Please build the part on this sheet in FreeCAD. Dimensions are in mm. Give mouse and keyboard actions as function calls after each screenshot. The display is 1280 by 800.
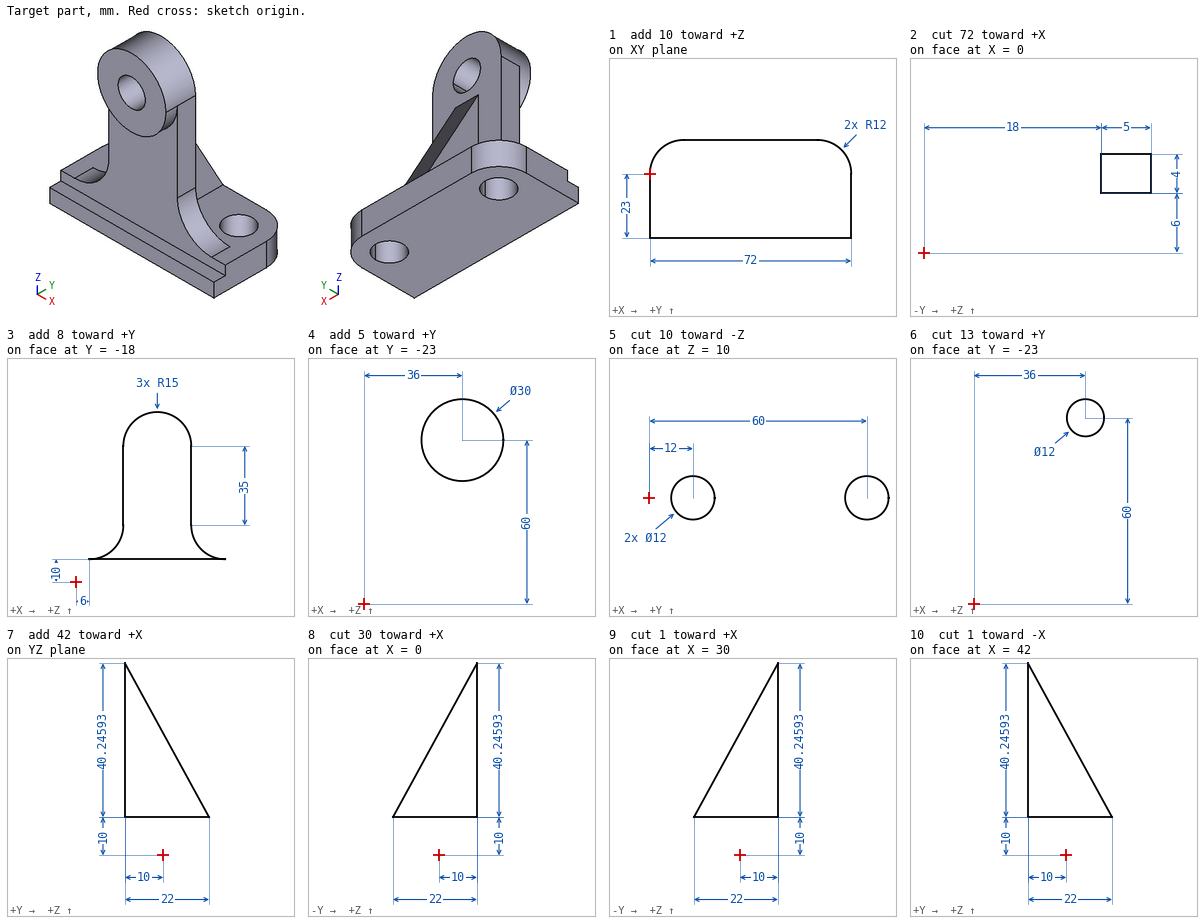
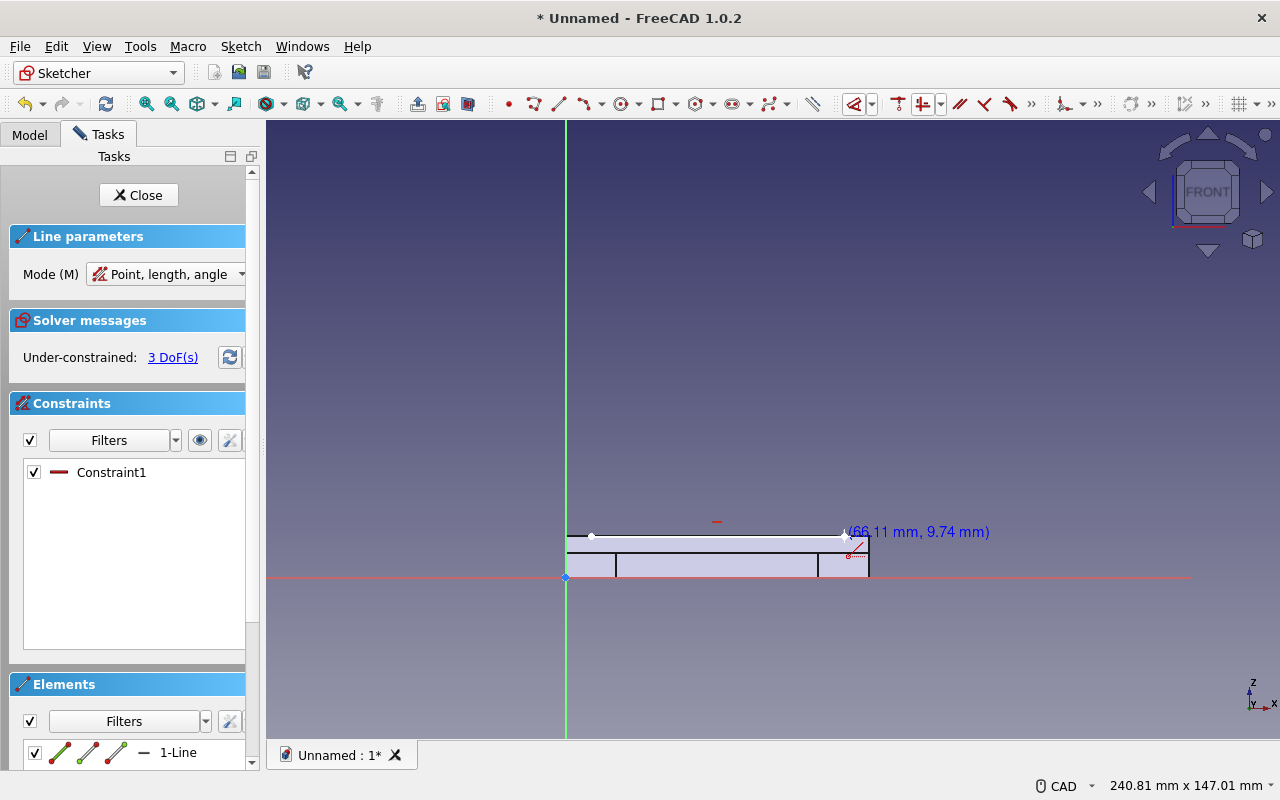
click(780, 473)
click(780, 325)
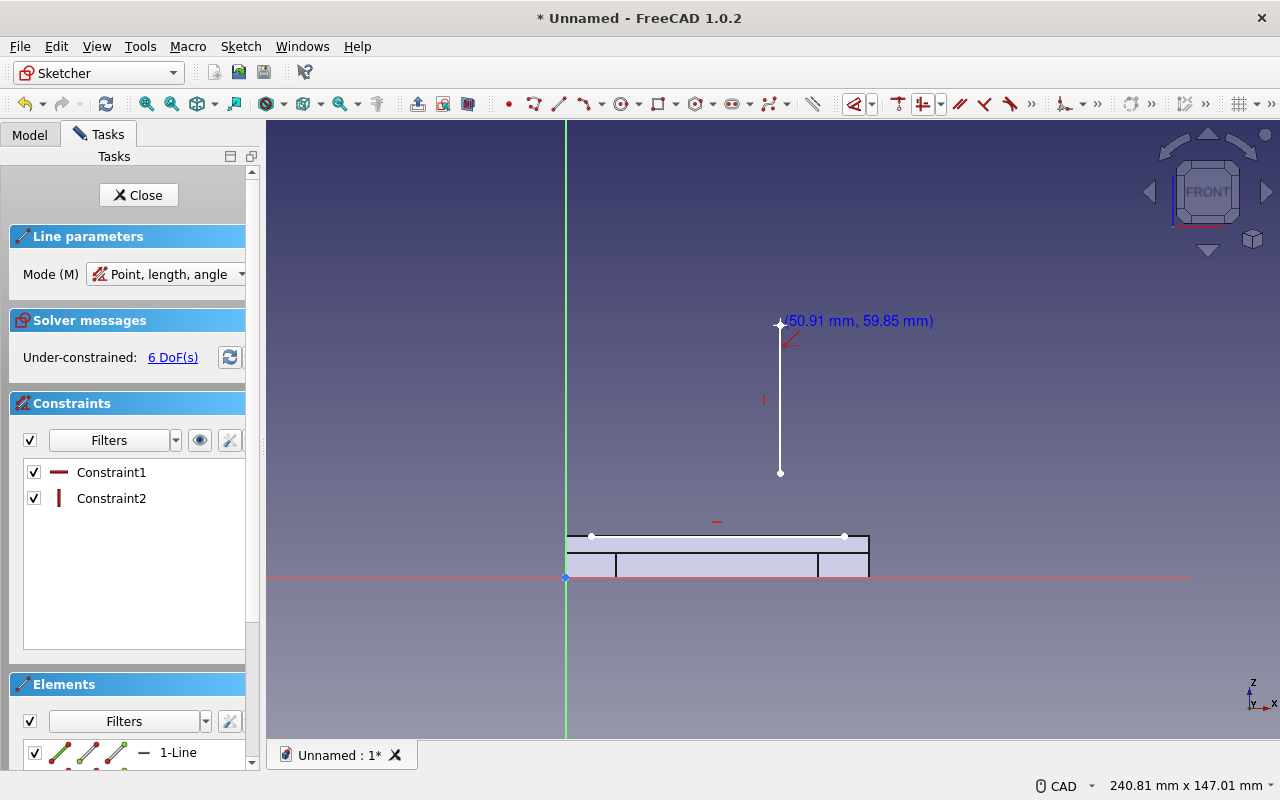
click(654, 325)
click(654, 473)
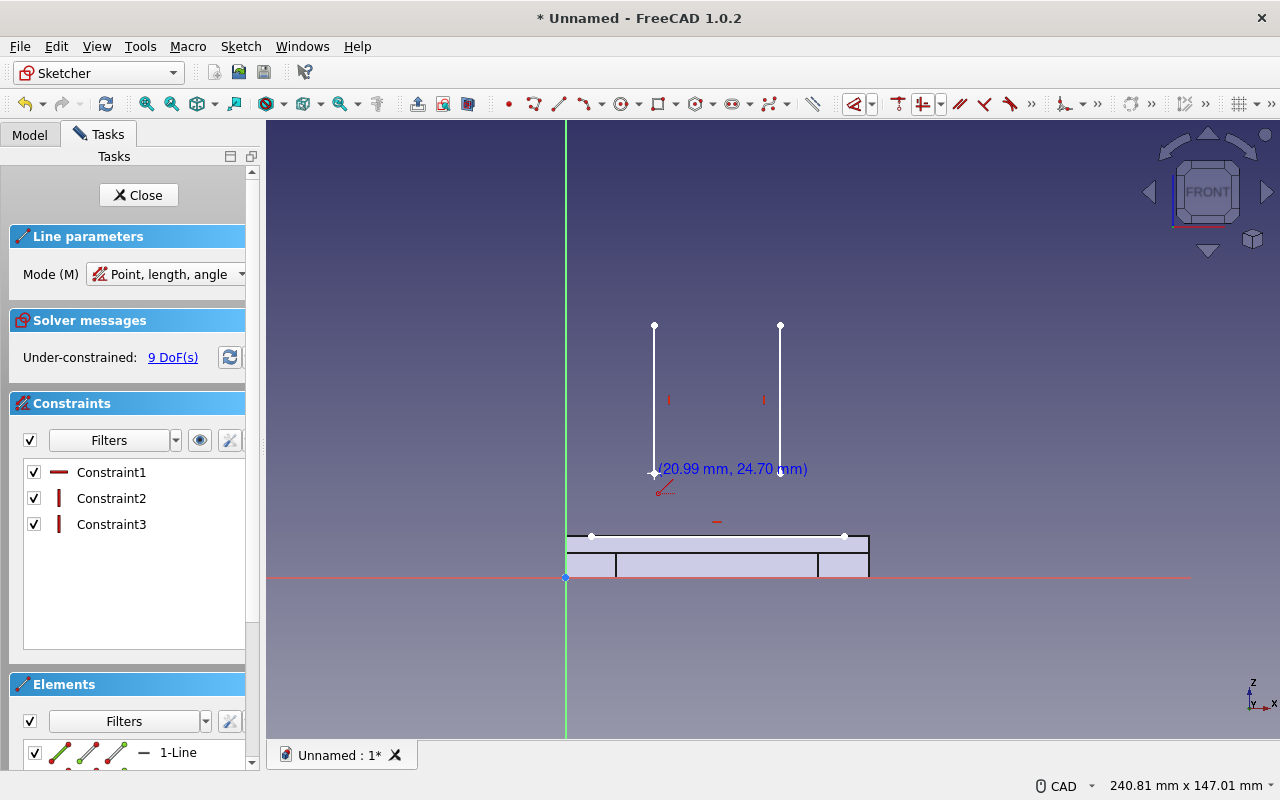
click(584, 104)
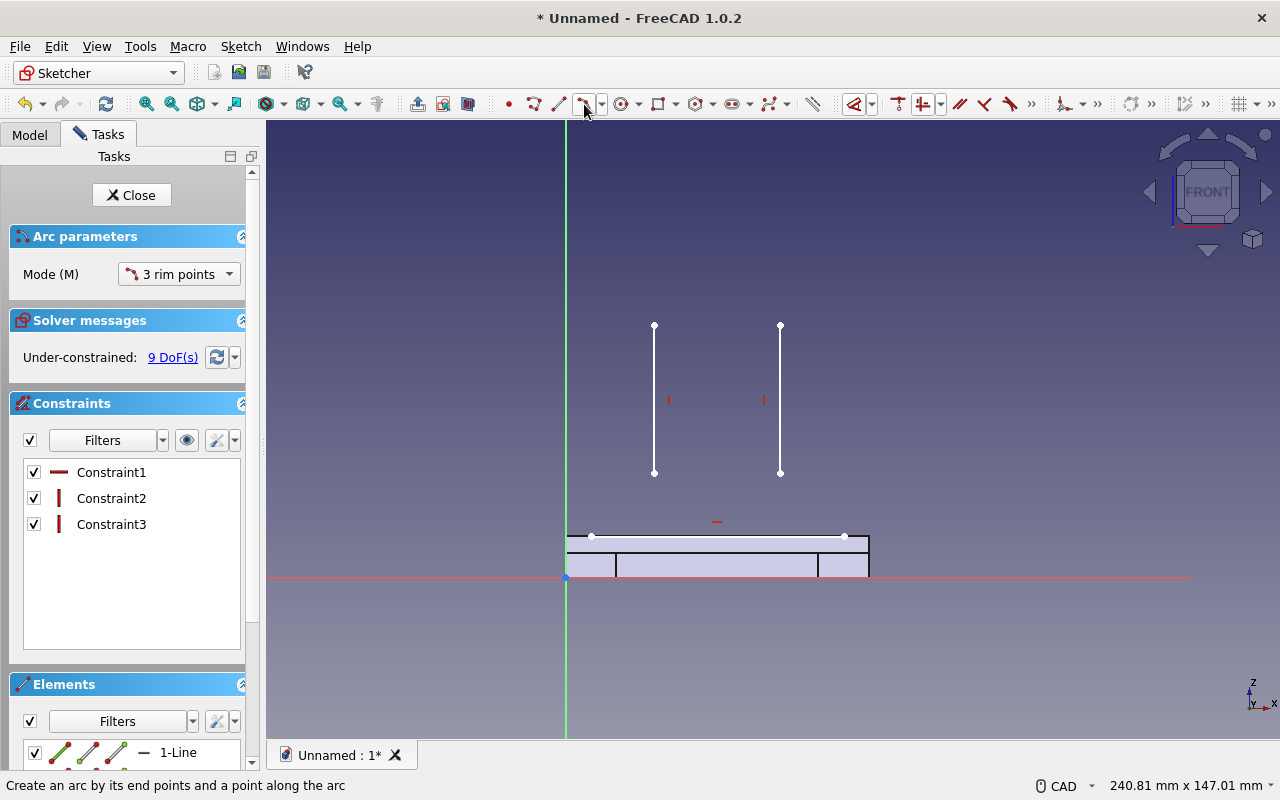
click(844, 537)
click(780, 474)
click(799, 517)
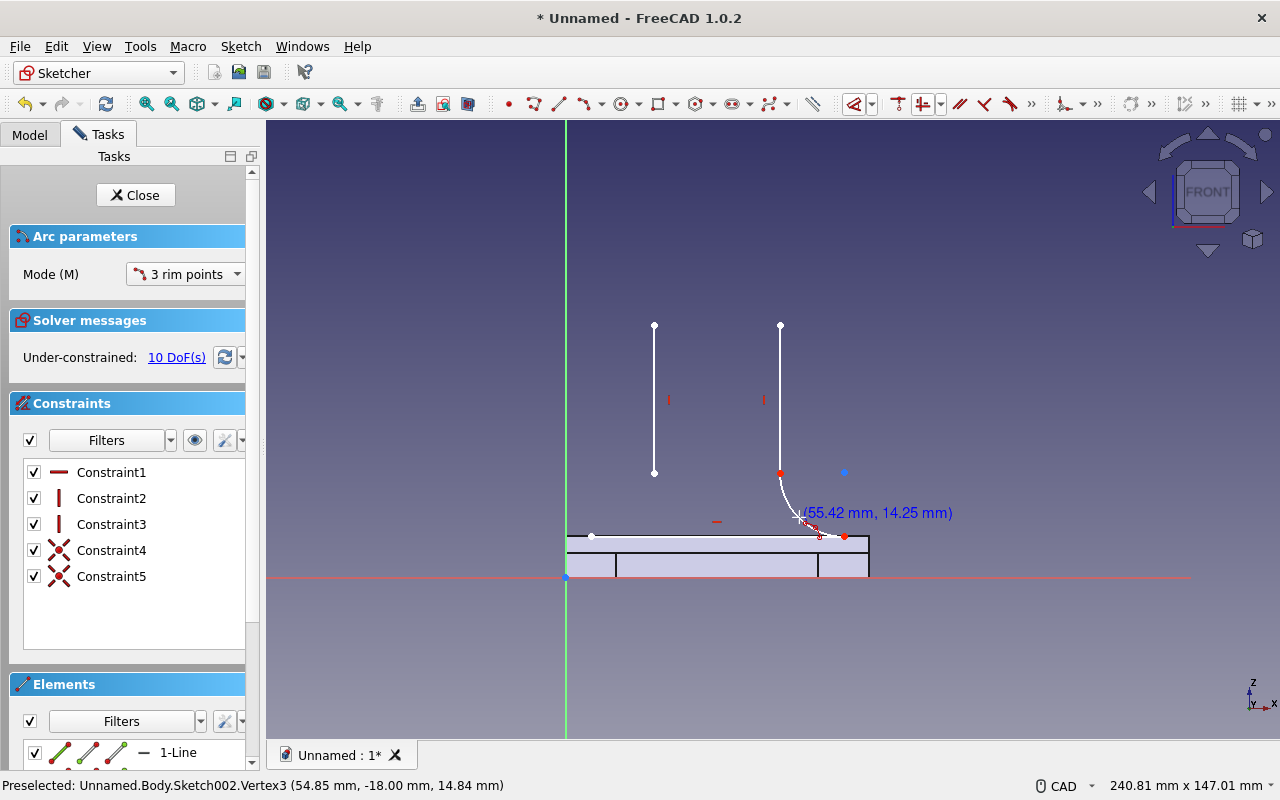
click(780, 326)
click(654, 326)
click(717, 262)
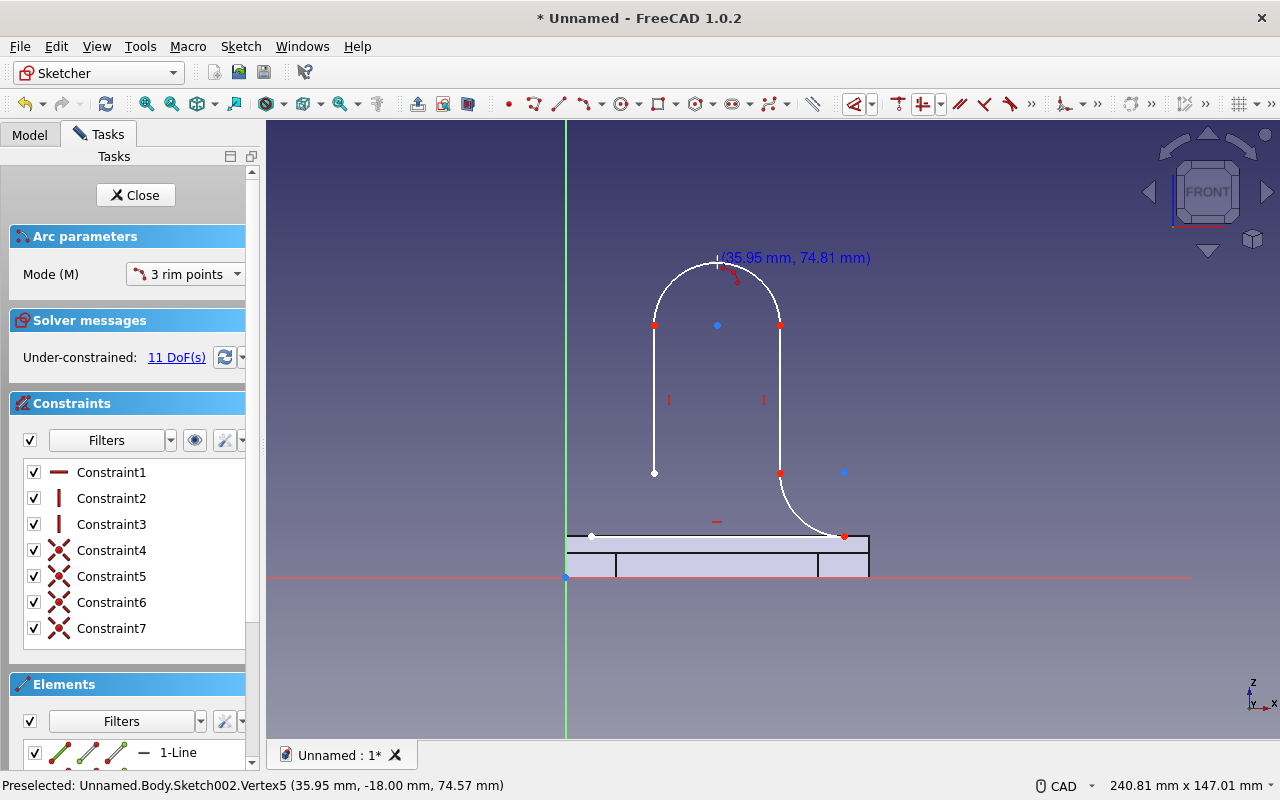
click(654, 474)
click(591, 537)
click(636, 517)
key(Escape)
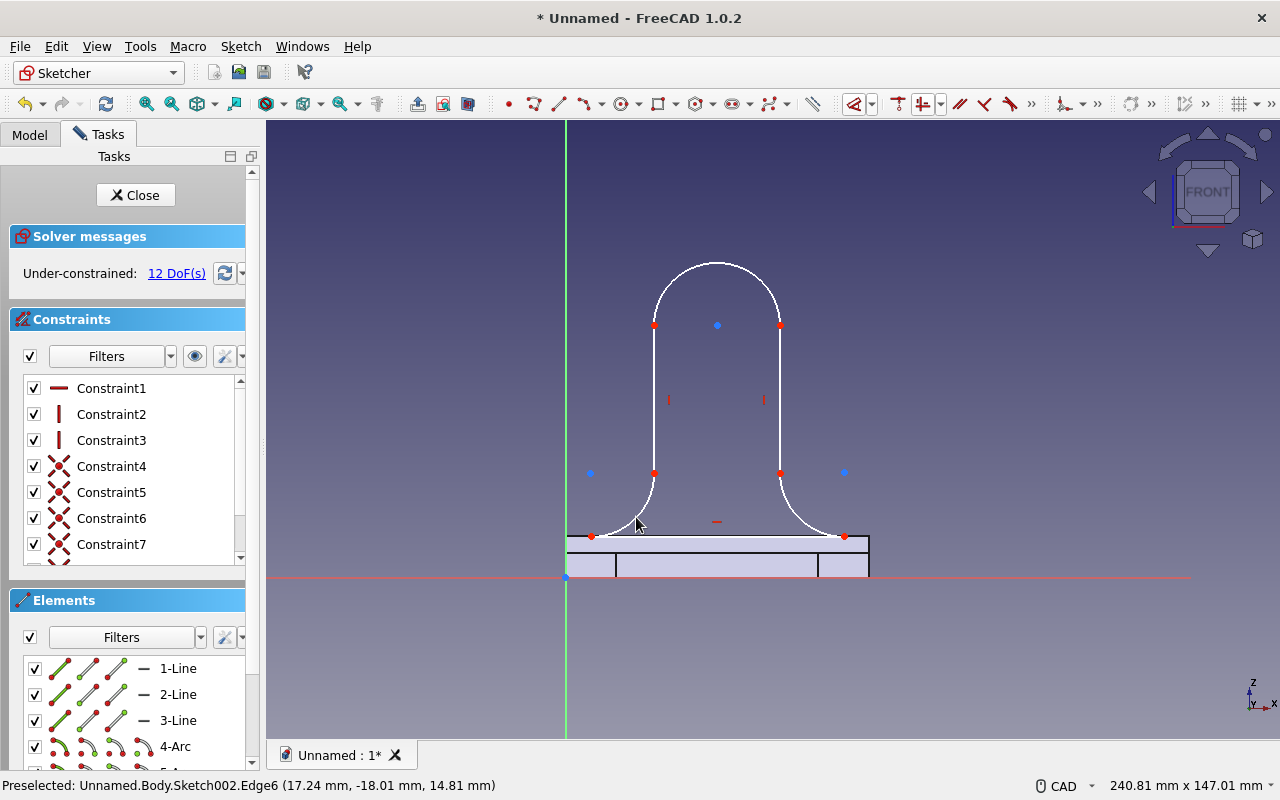
click(667, 537)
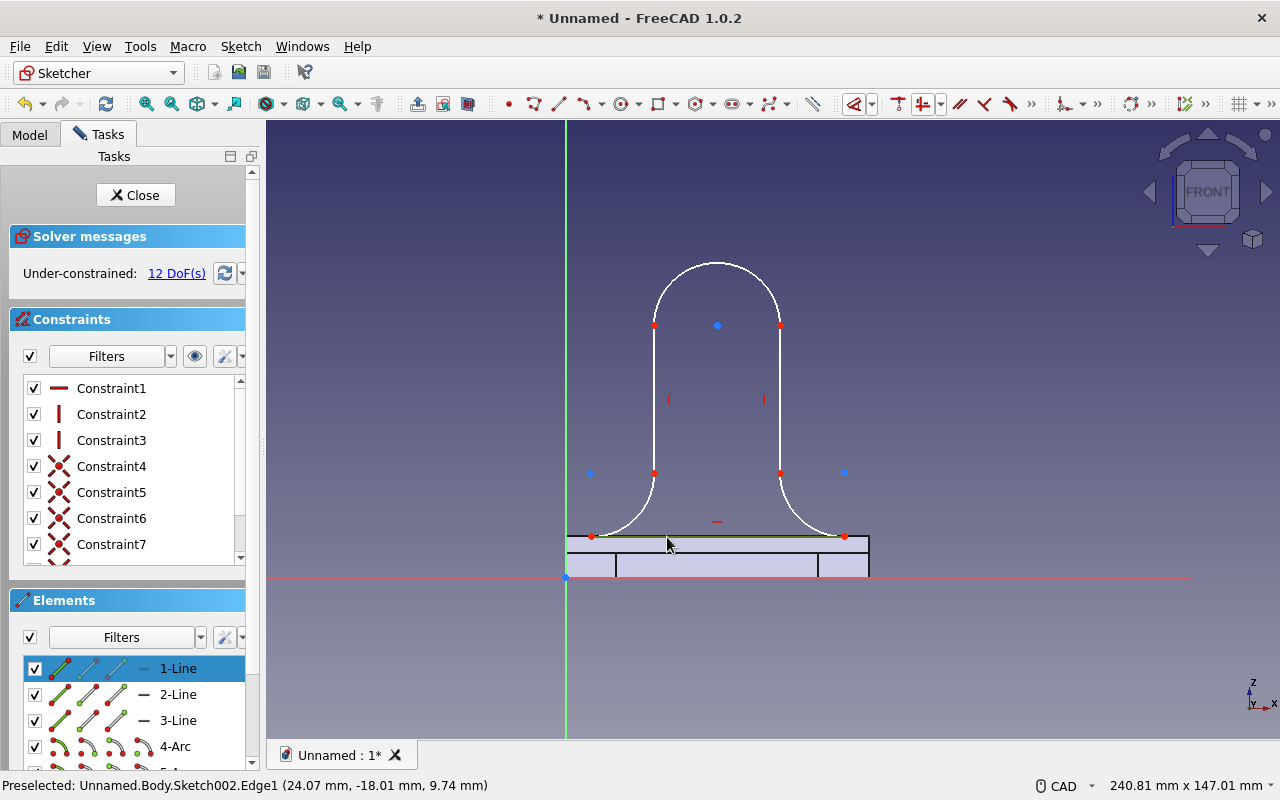
click(788, 503)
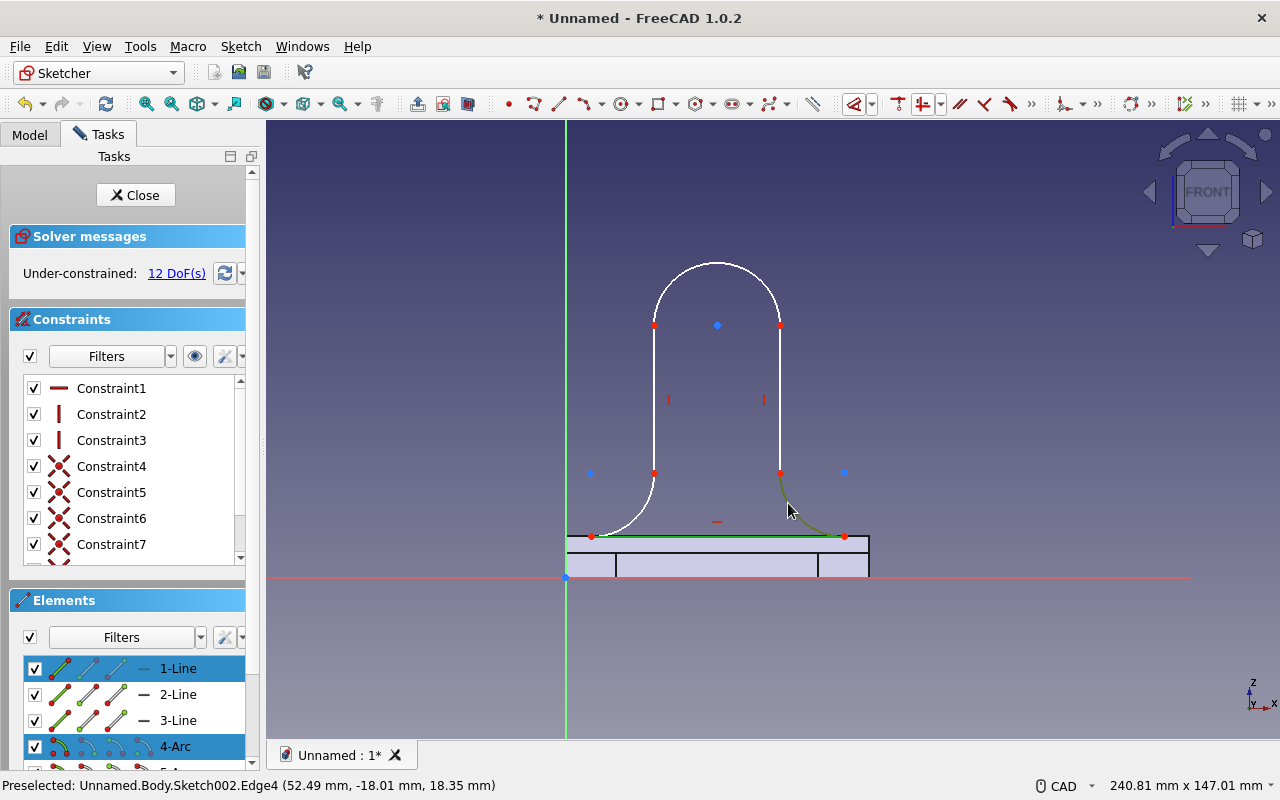
key(t)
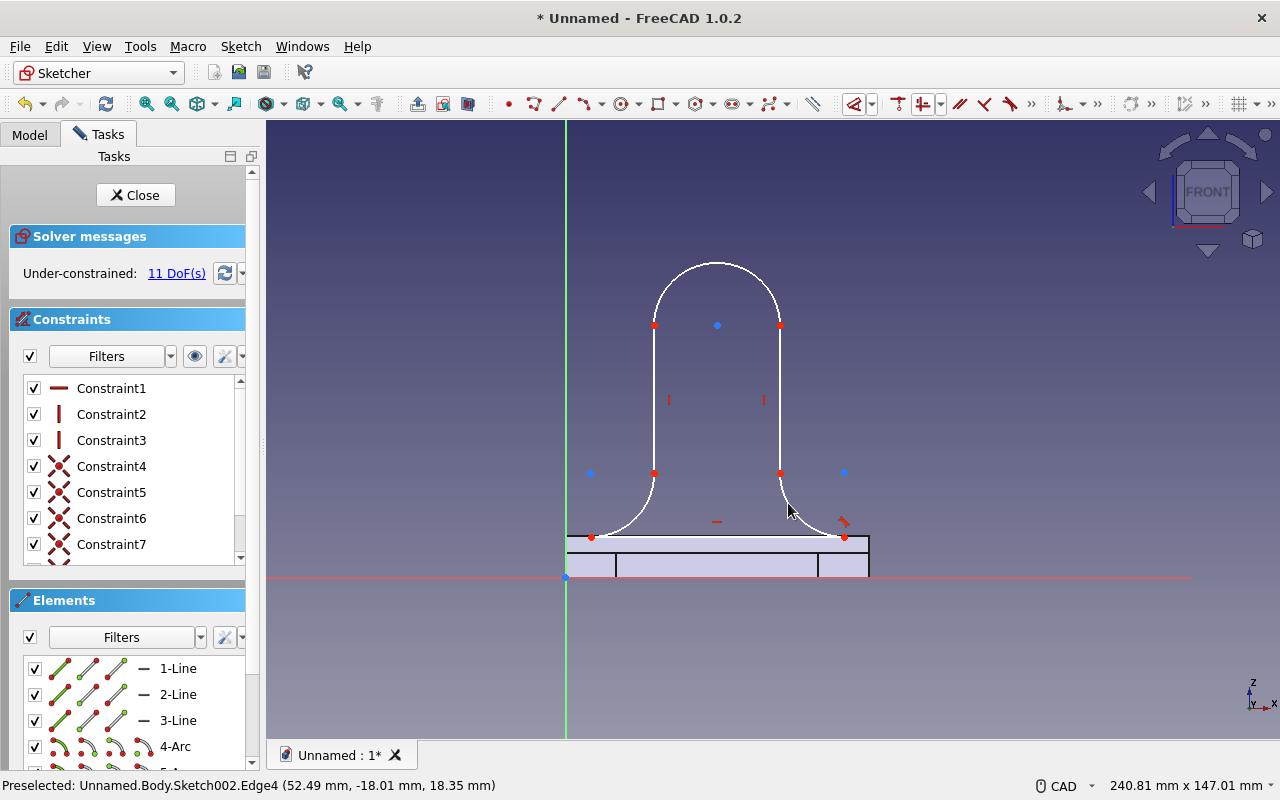
click(667, 537)